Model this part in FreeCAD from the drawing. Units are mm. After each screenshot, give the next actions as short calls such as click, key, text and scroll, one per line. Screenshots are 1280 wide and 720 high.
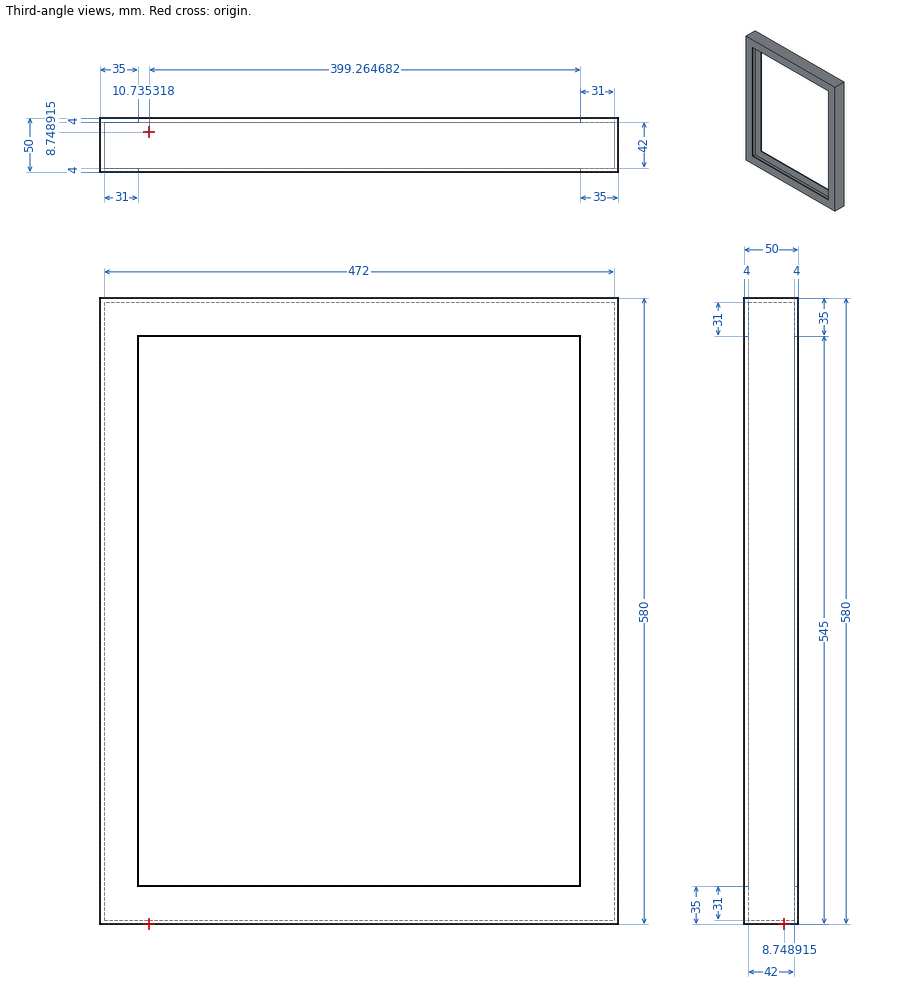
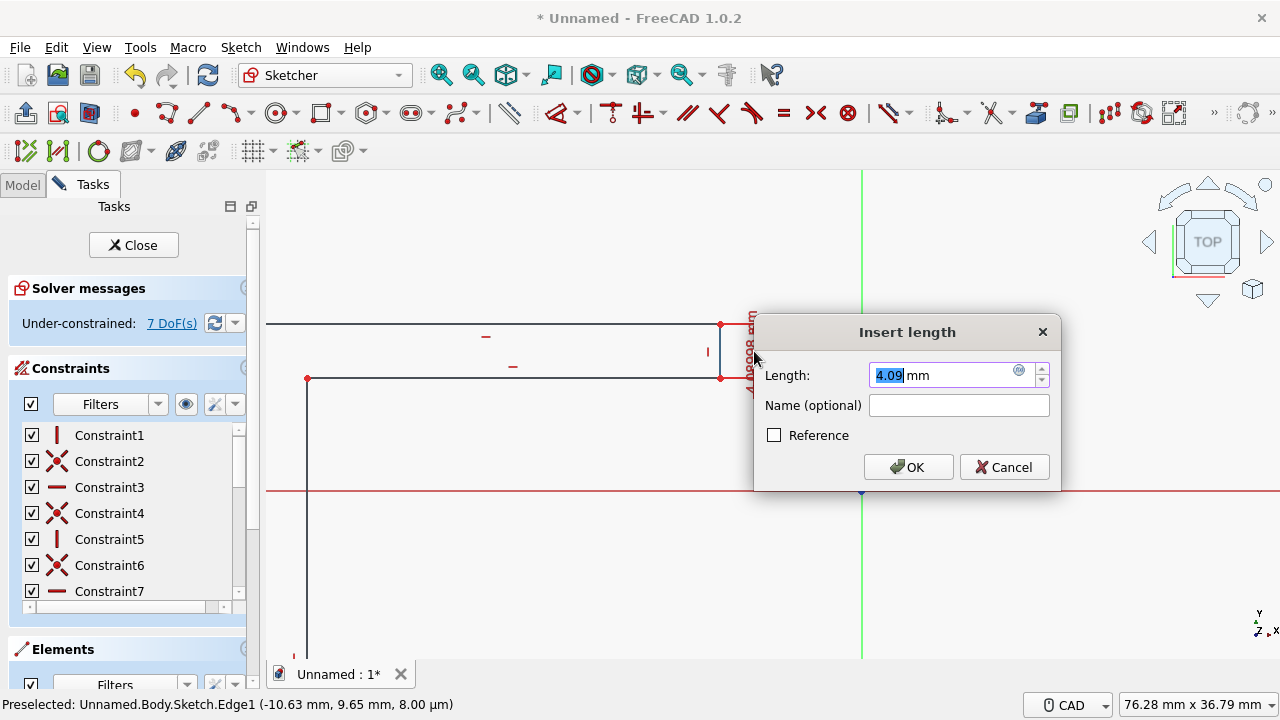
text(4)
key(Return)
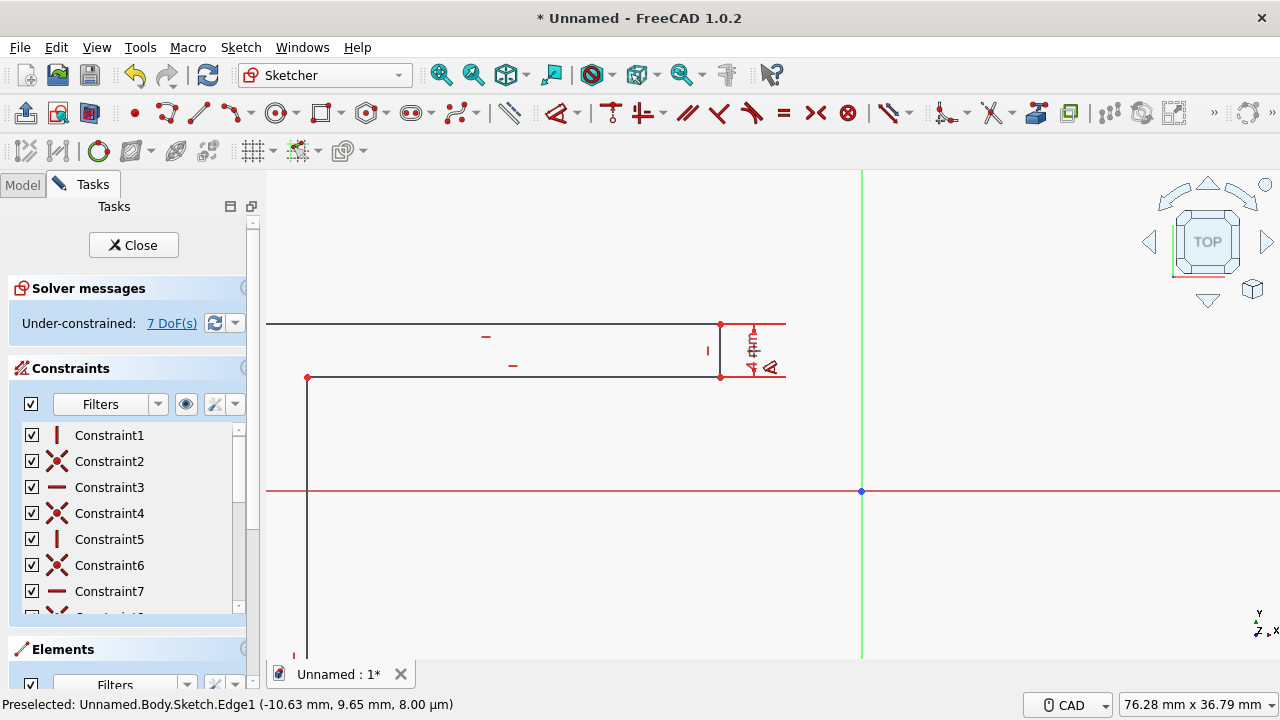
scroll(824, 219, down, 4)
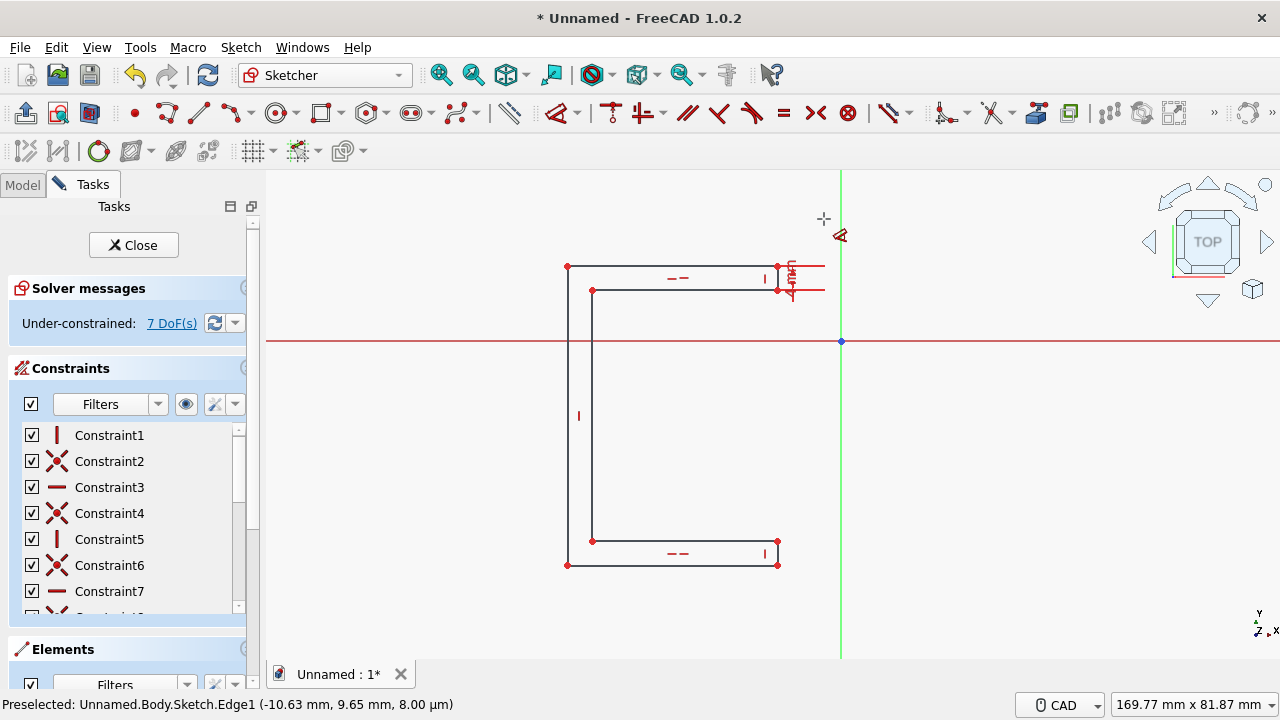
scroll(778, 558, up, 4)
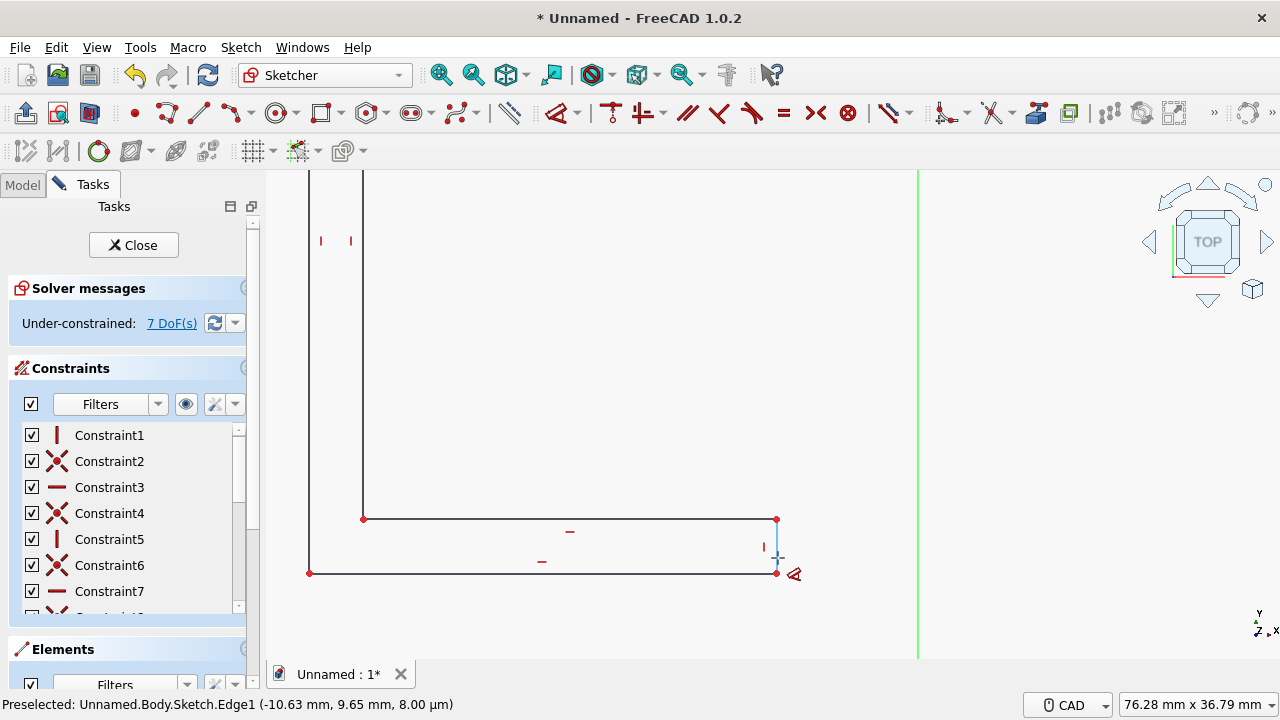
click(777, 557)
click(811, 547)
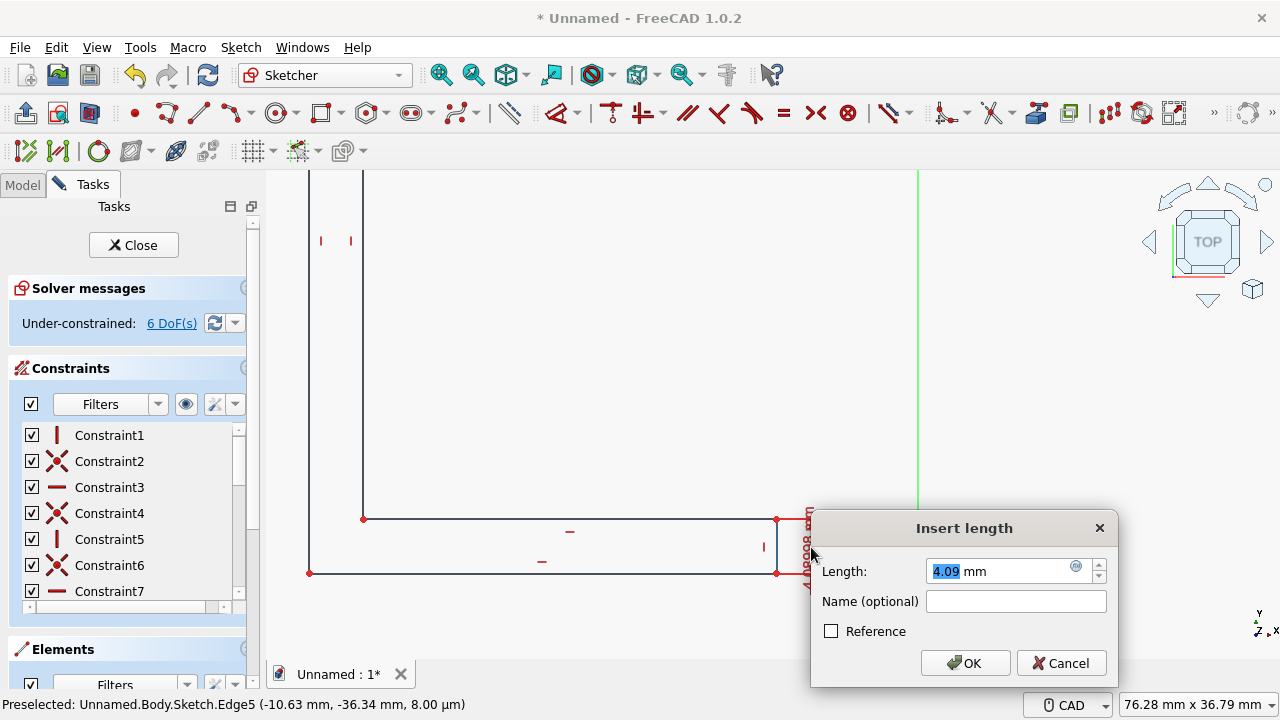
text(4)
key(Return)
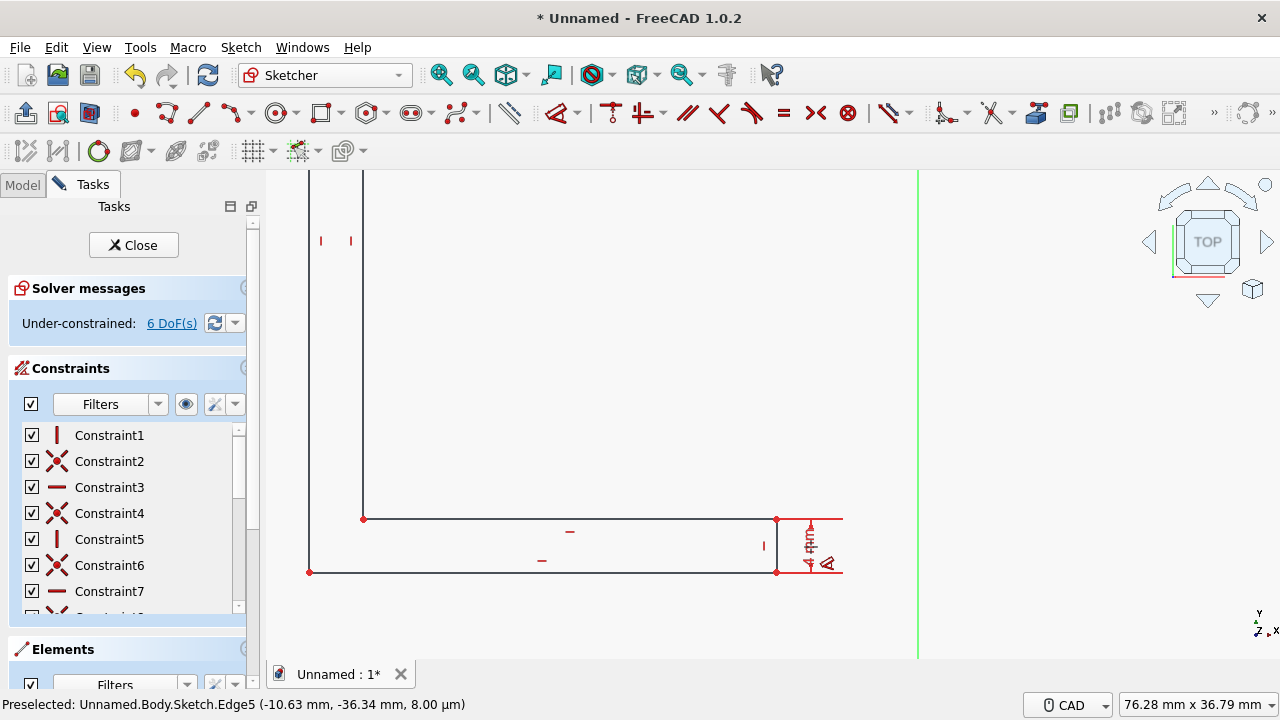
scroll(778, 559, down, 4)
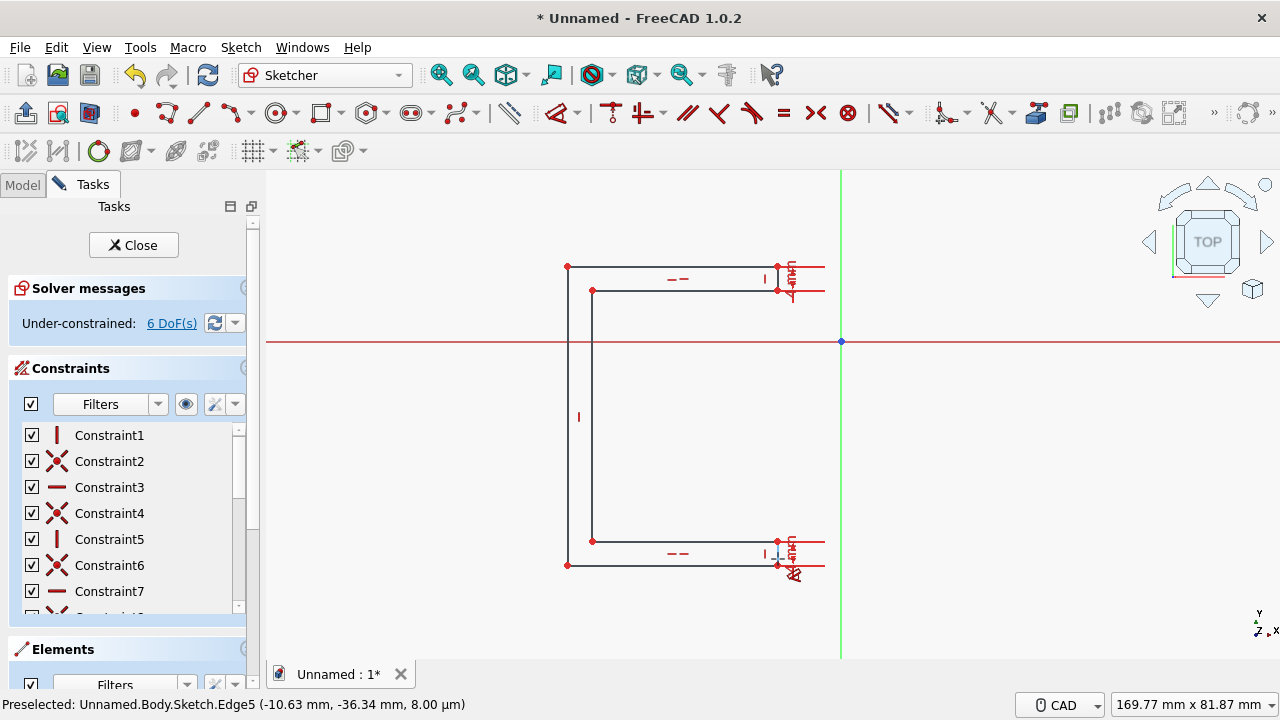
click(715, 267)
click(673, 233)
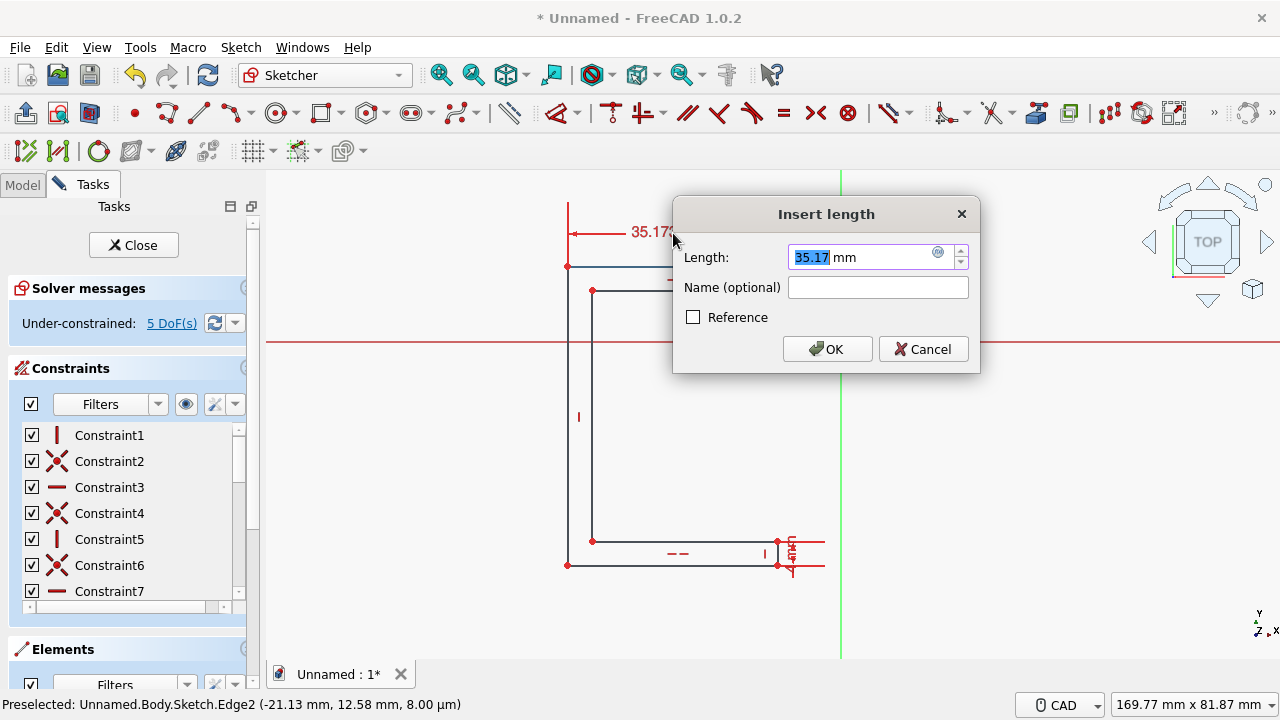
text(35)
key(Return)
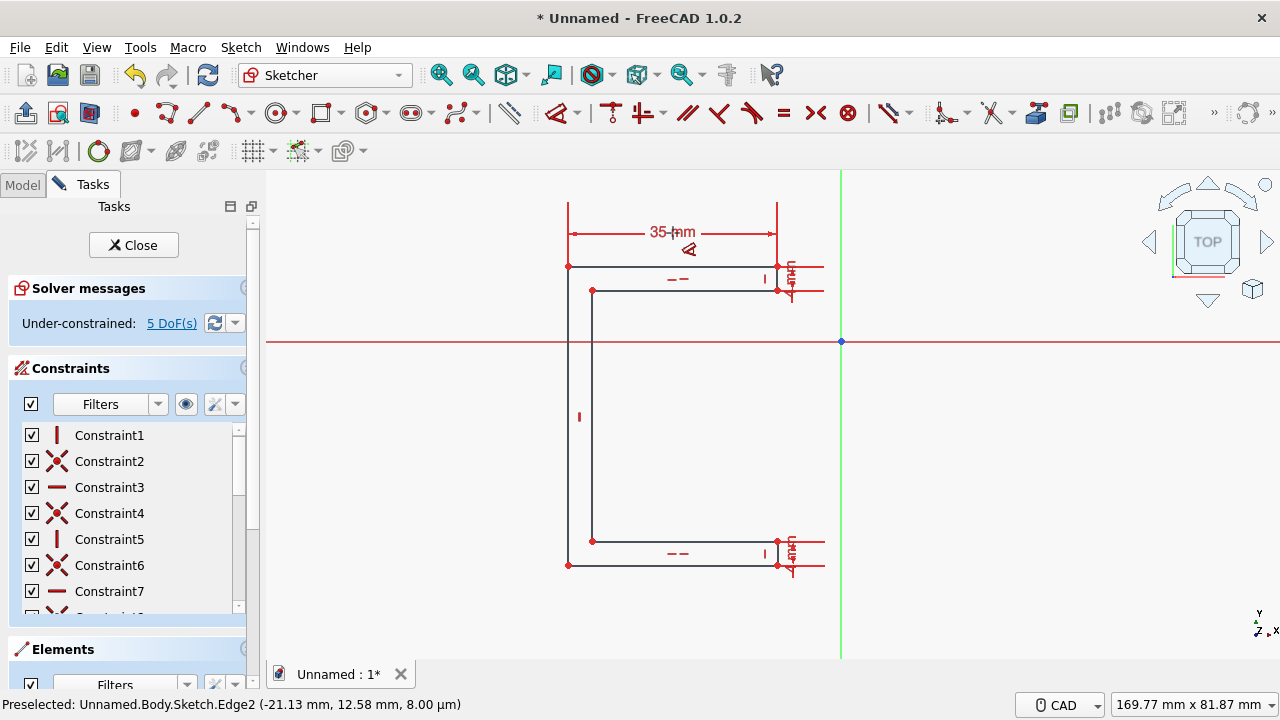
click(568, 356)
click(534, 416)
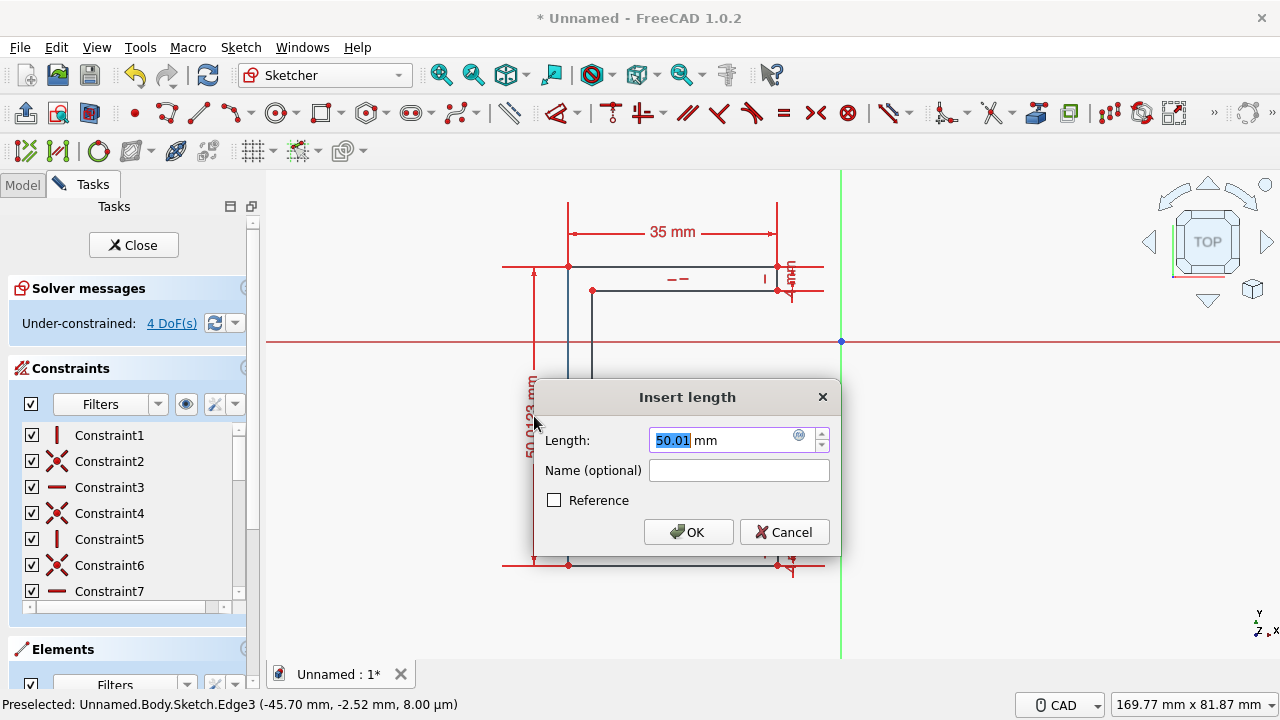
text(50)
key(Return)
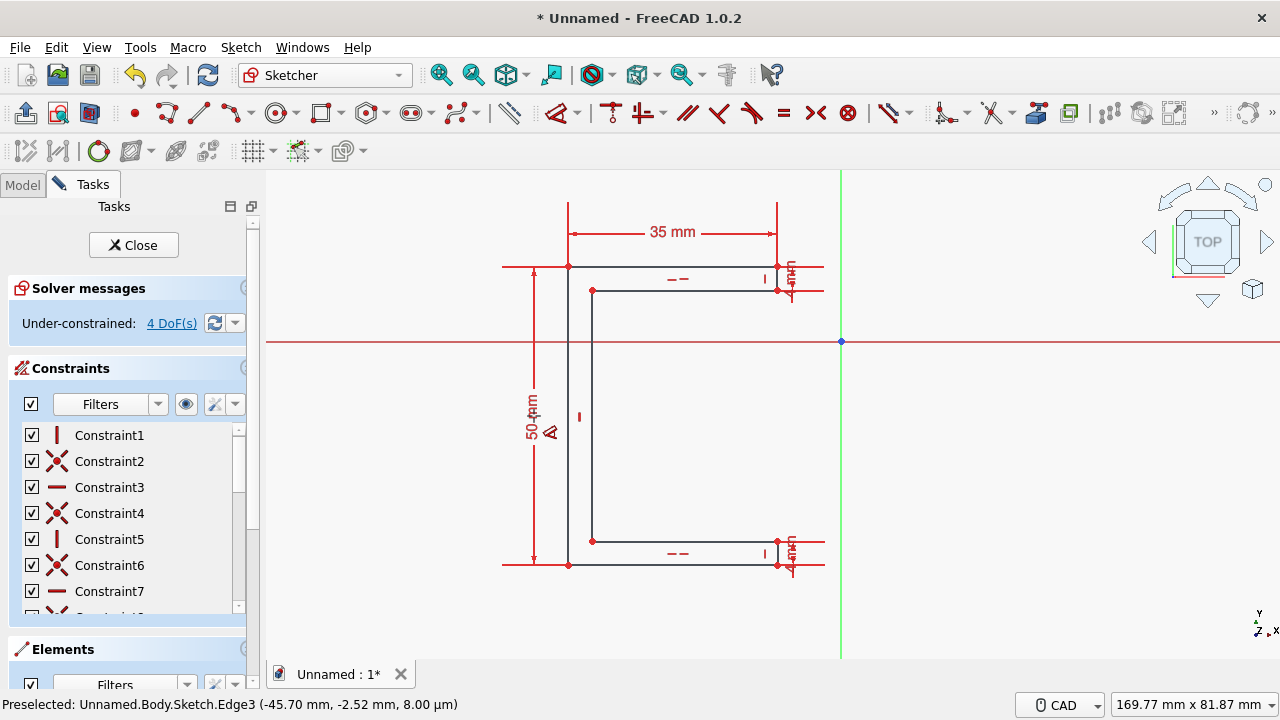
click(631, 565)
click(673, 599)